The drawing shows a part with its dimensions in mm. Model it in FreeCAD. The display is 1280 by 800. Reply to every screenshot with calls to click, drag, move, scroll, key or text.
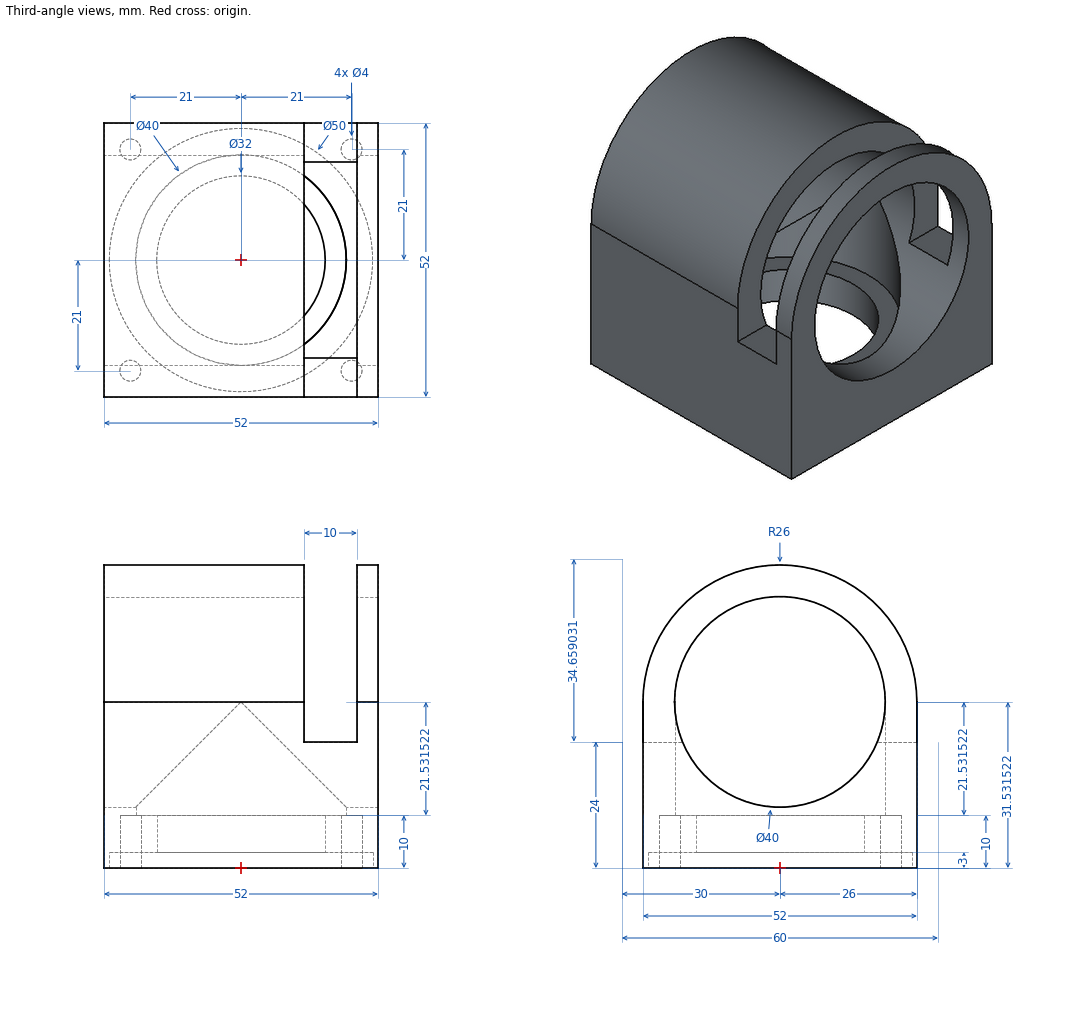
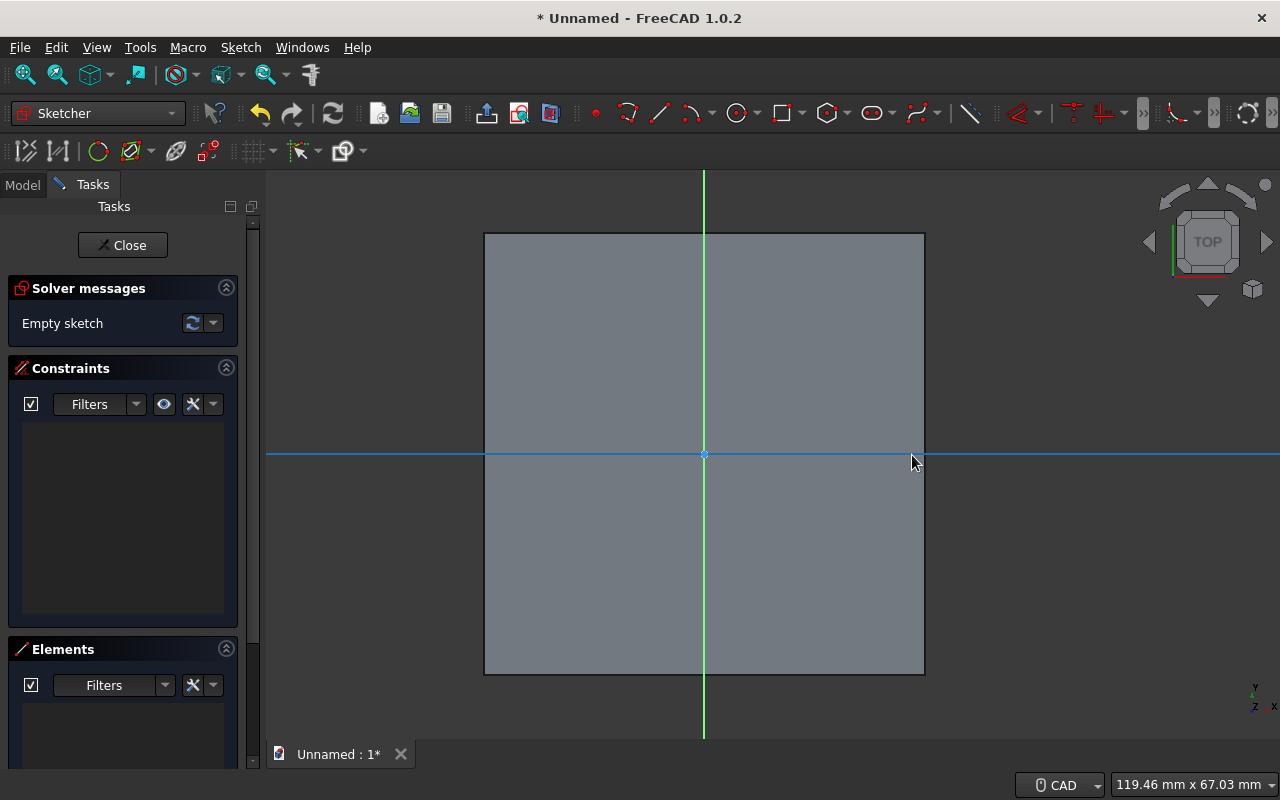
click(738, 114)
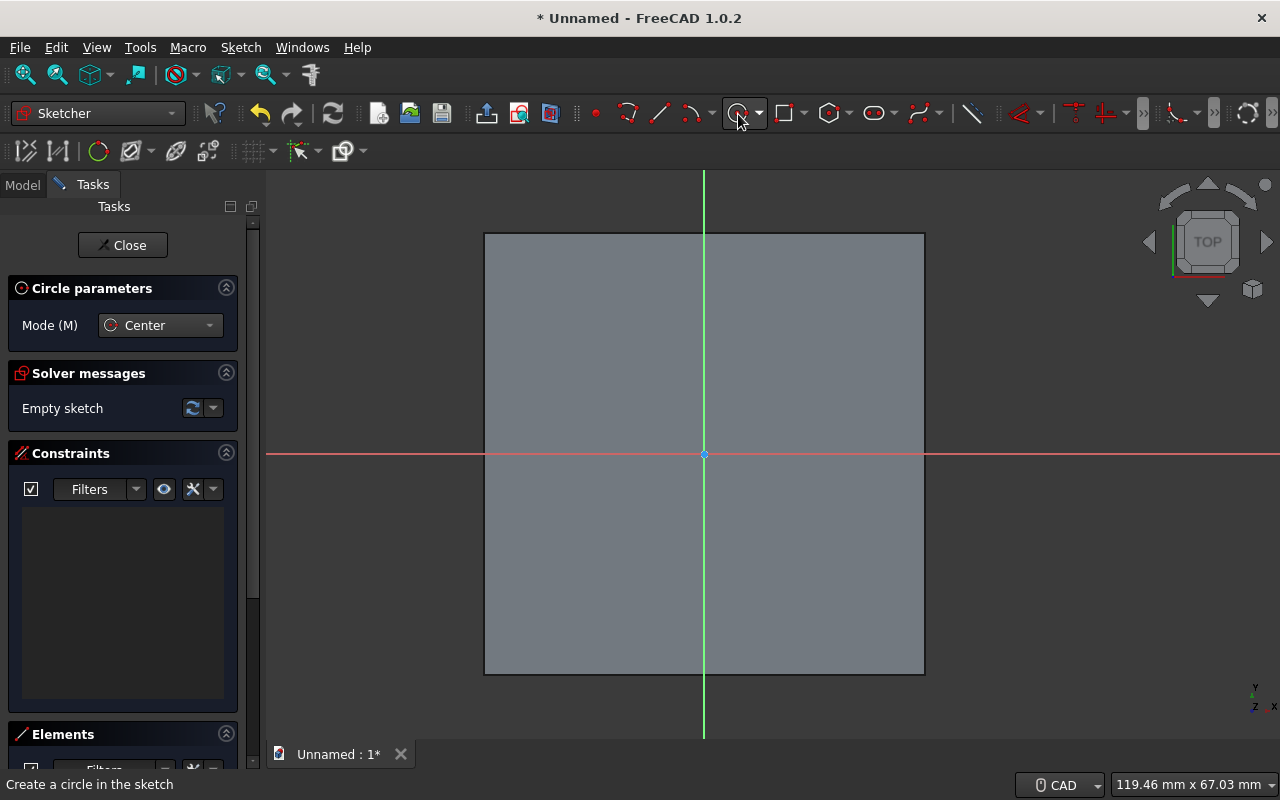
scroll(883, 276, up, 2)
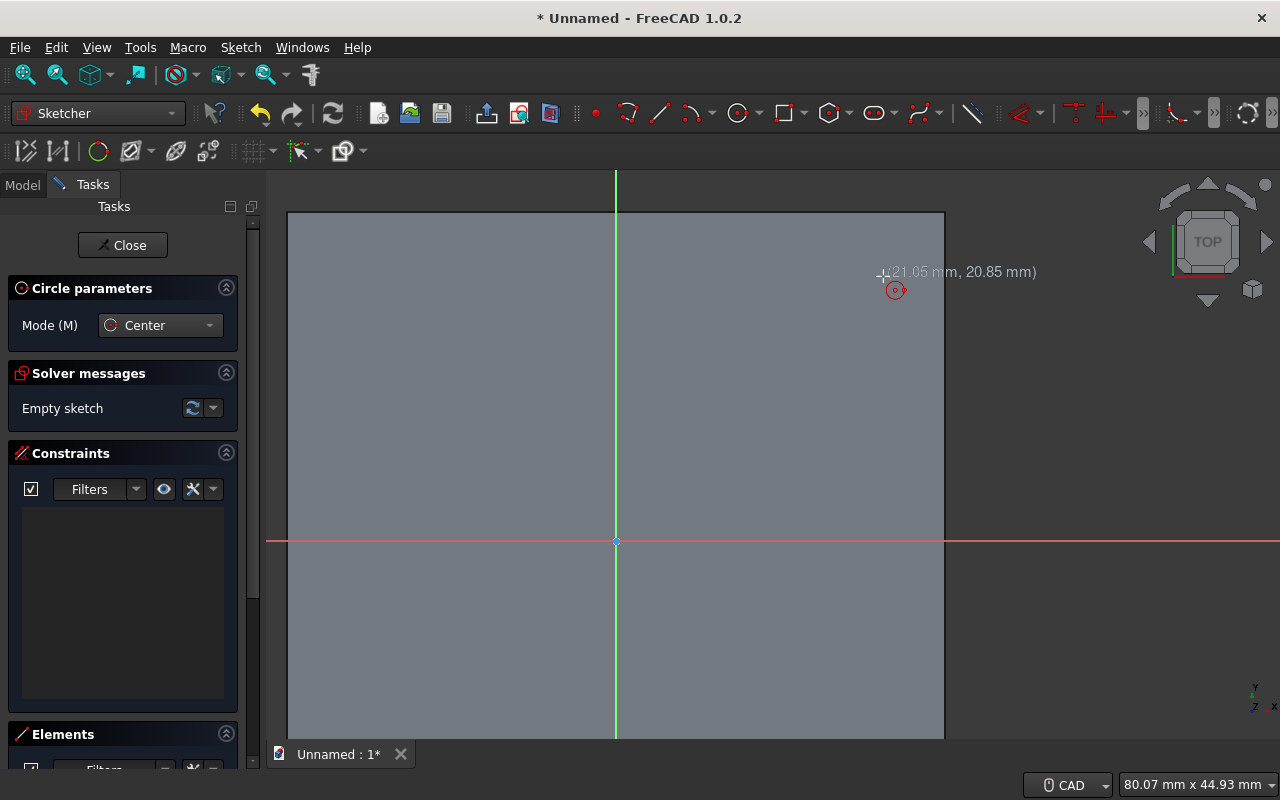
click(882, 276)
click(900, 258)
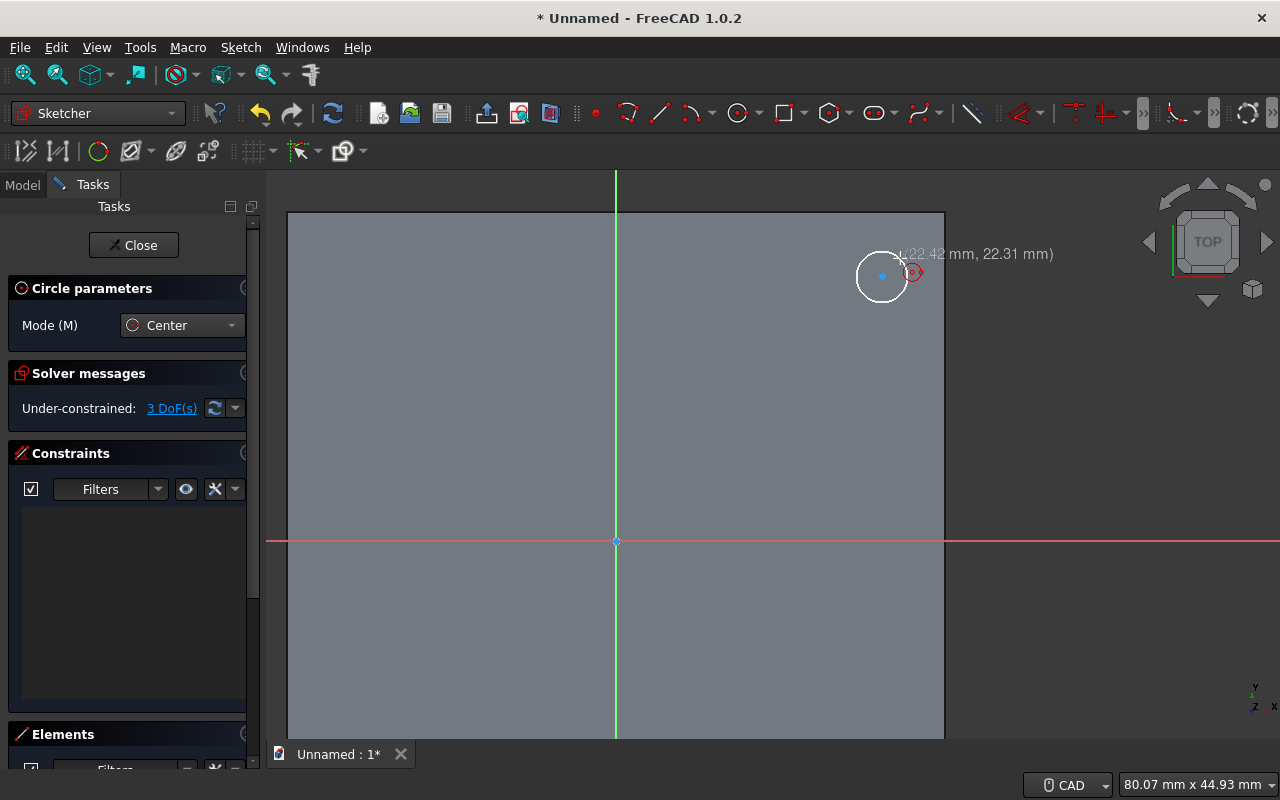
click(350, 276)
click(368, 258)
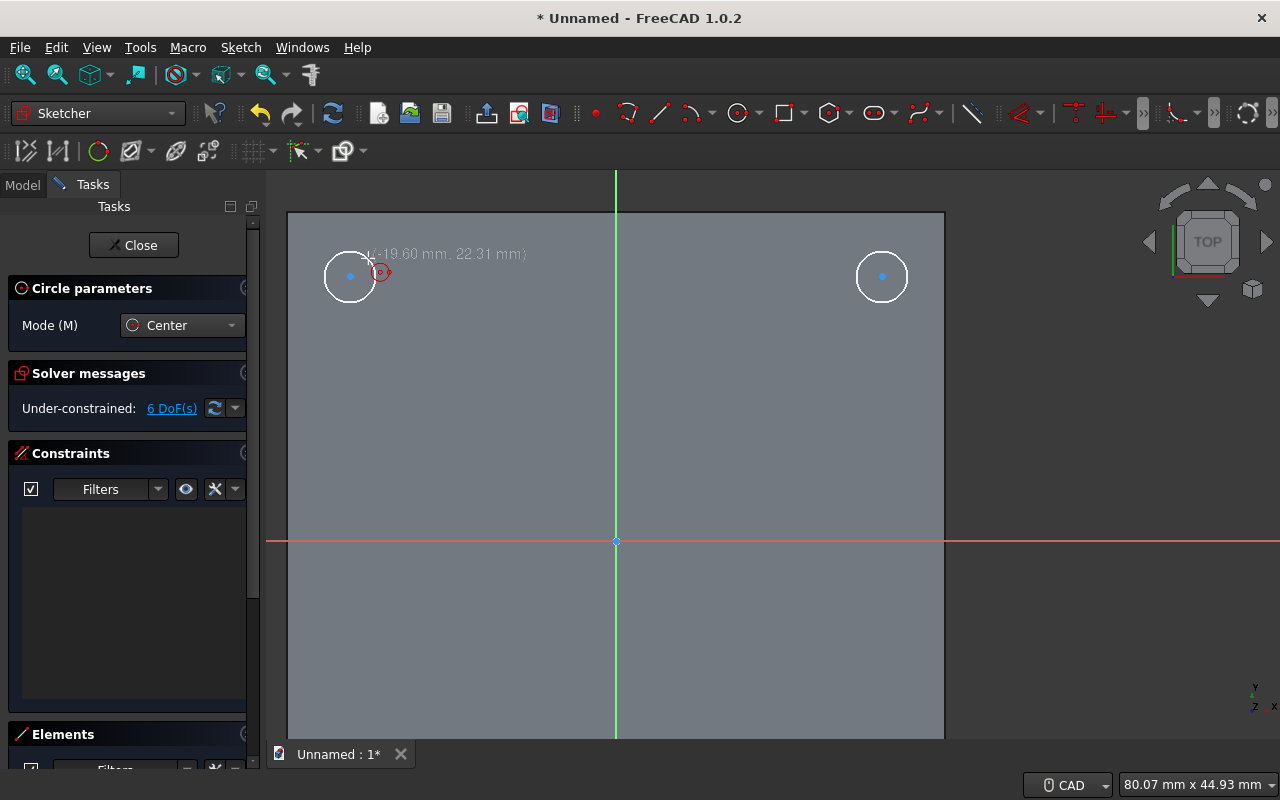
scroll(884, 278, down, 2)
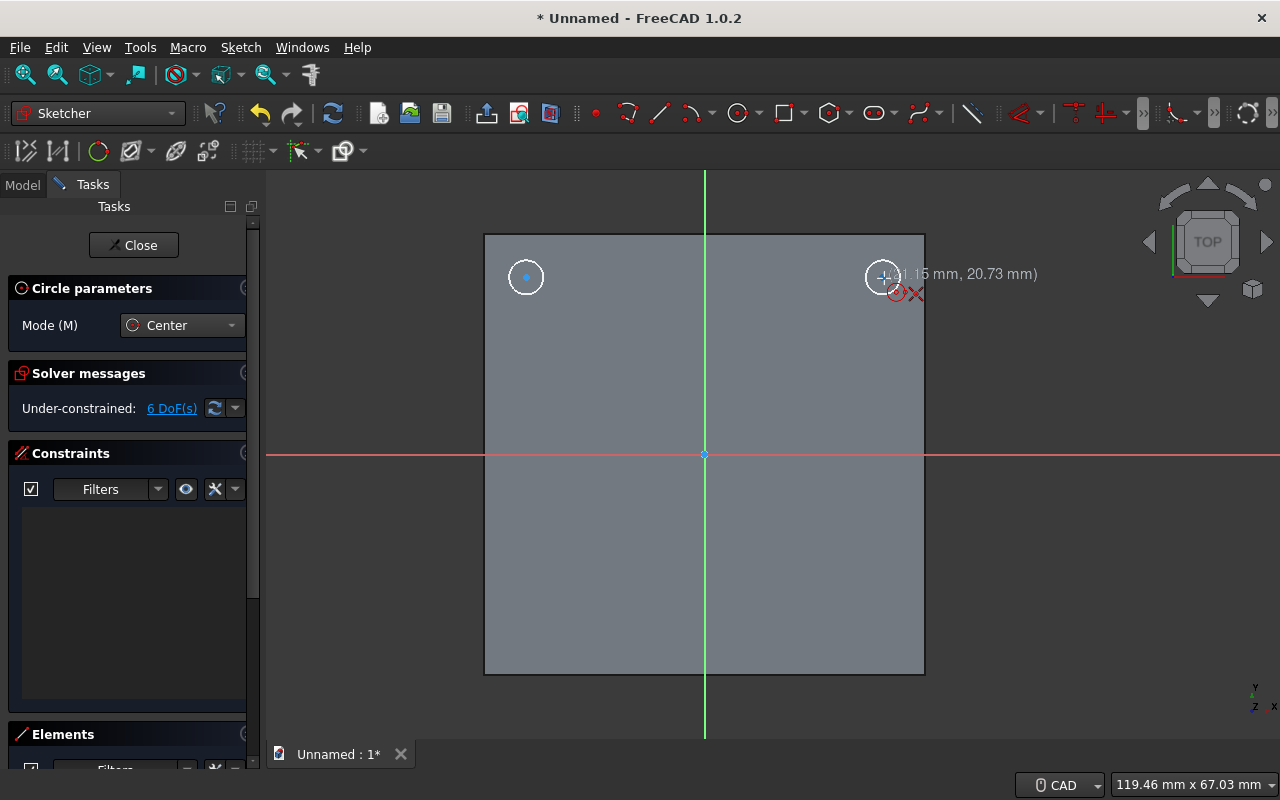
scroll(526, 633, up, 2)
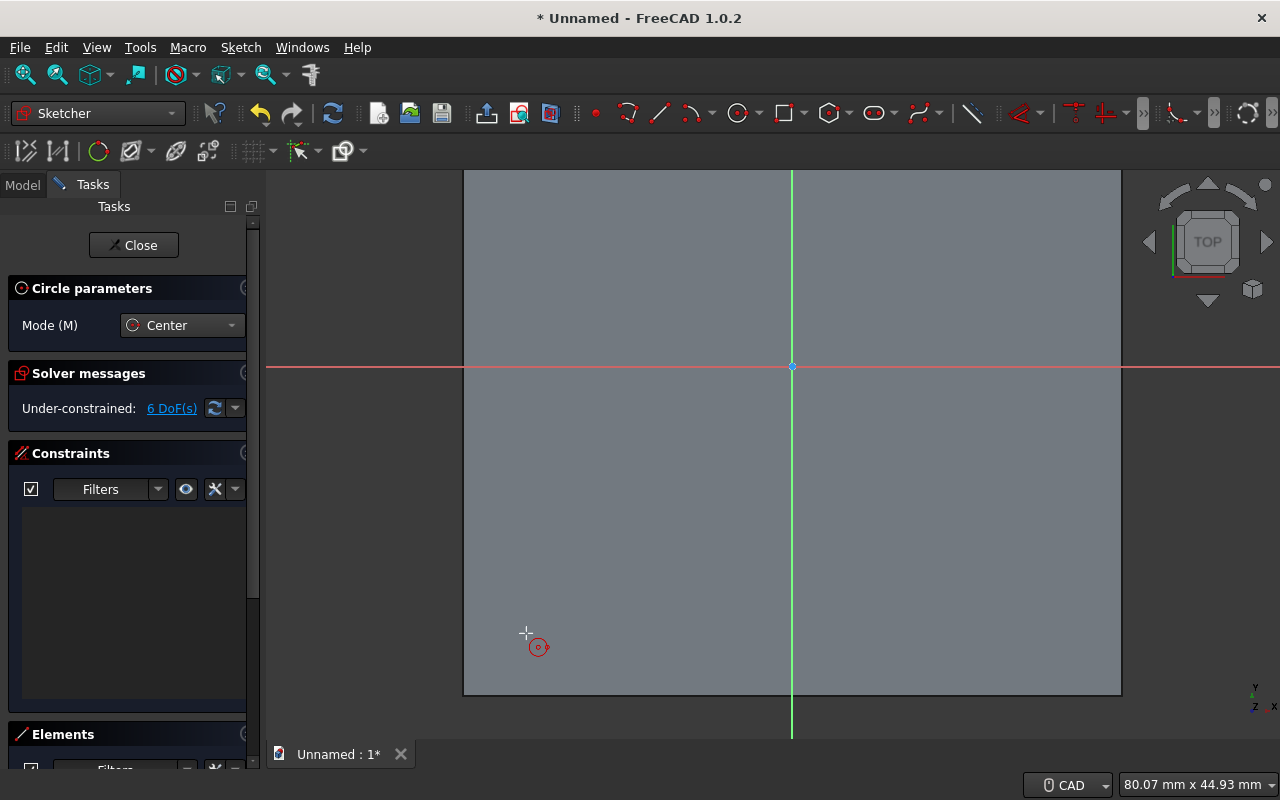
click(526, 632)
click(544, 615)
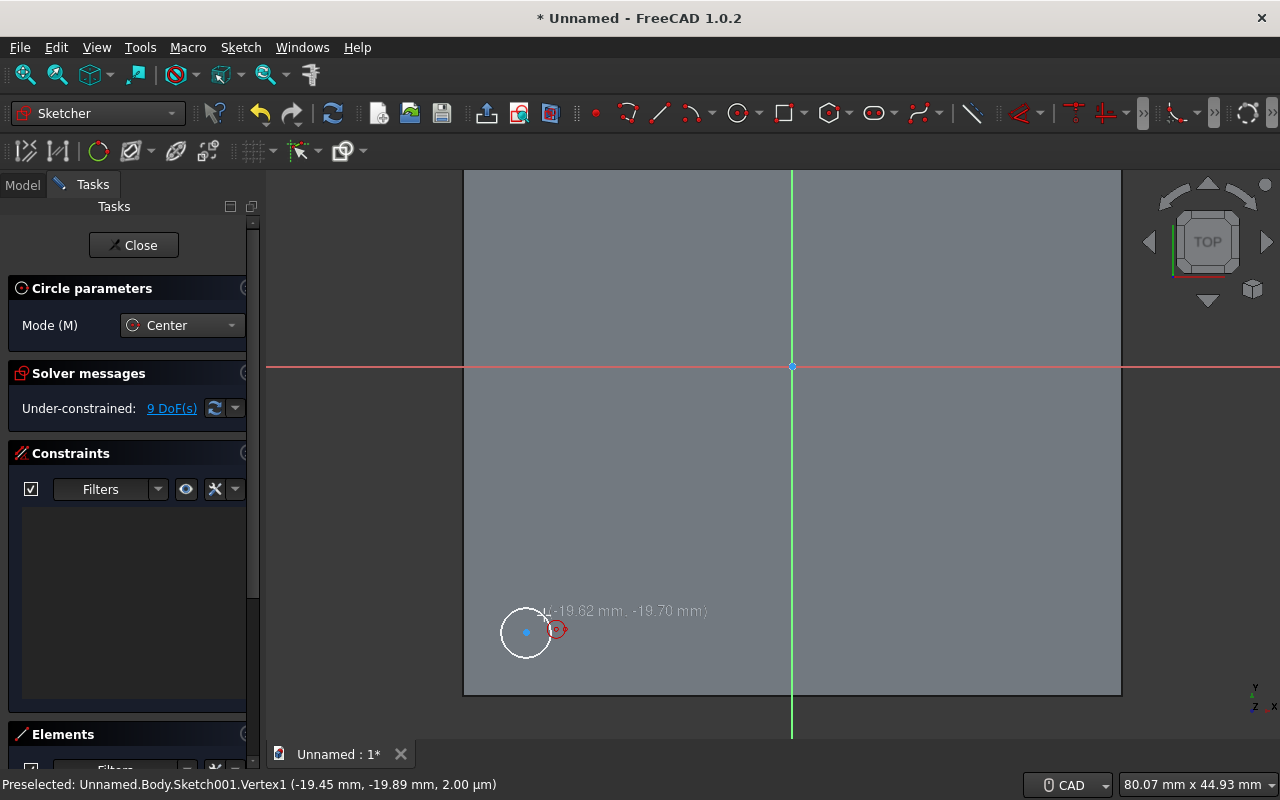
click(1058, 632)
click(1076, 615)
key(Escape)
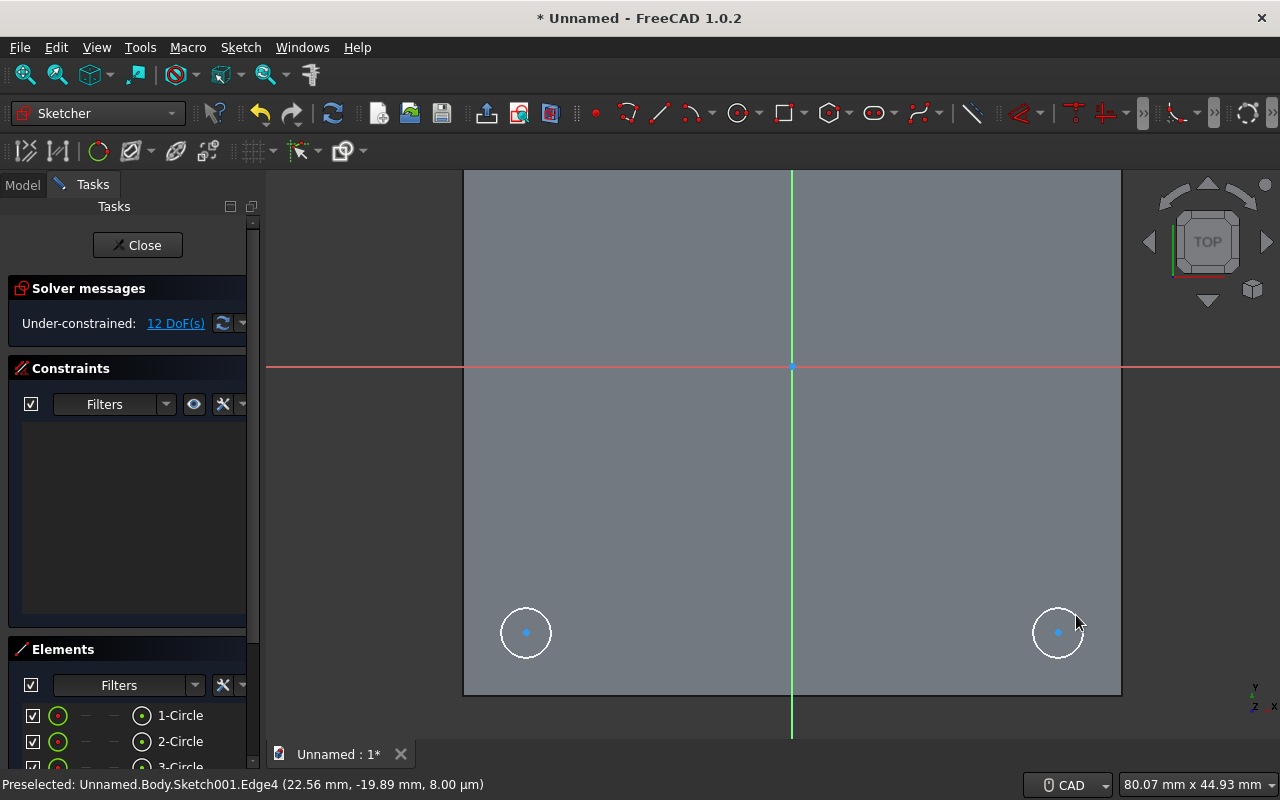
scroll(526, 633, down, 2)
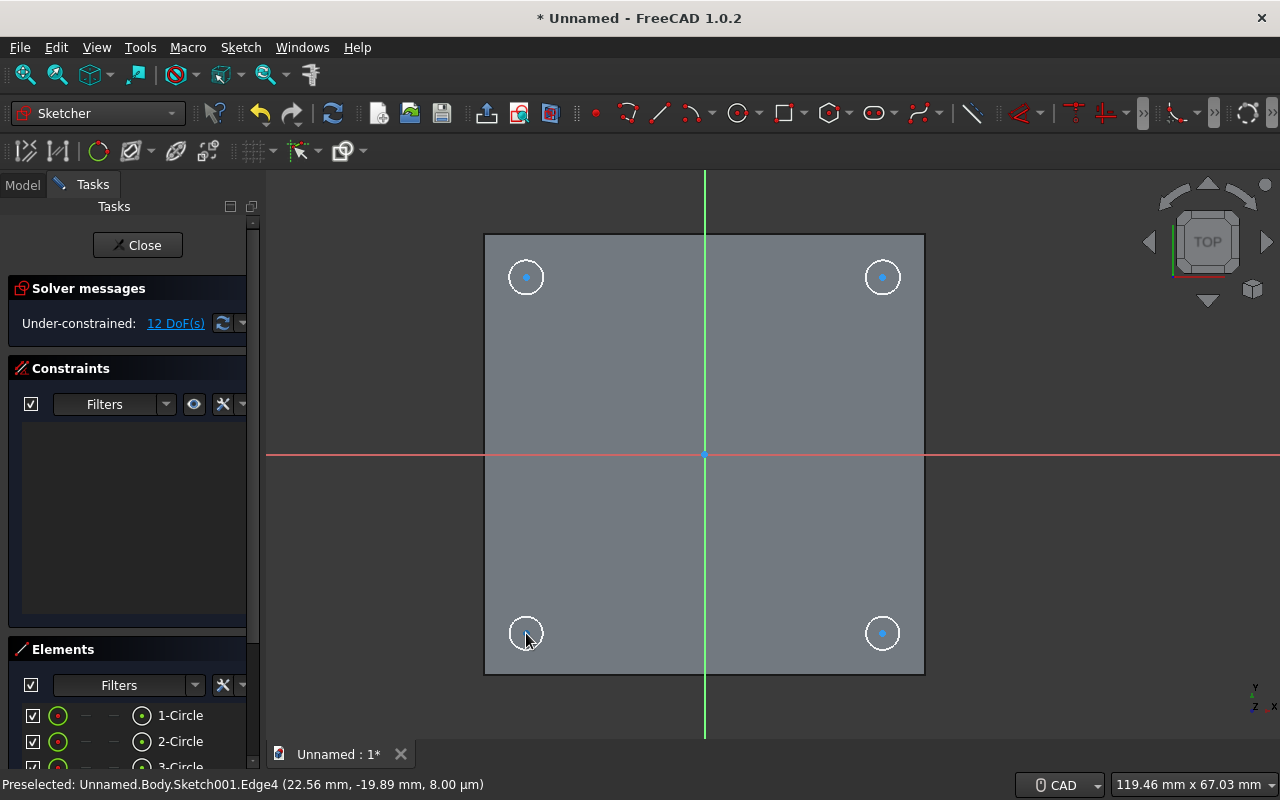
click(895, 265)